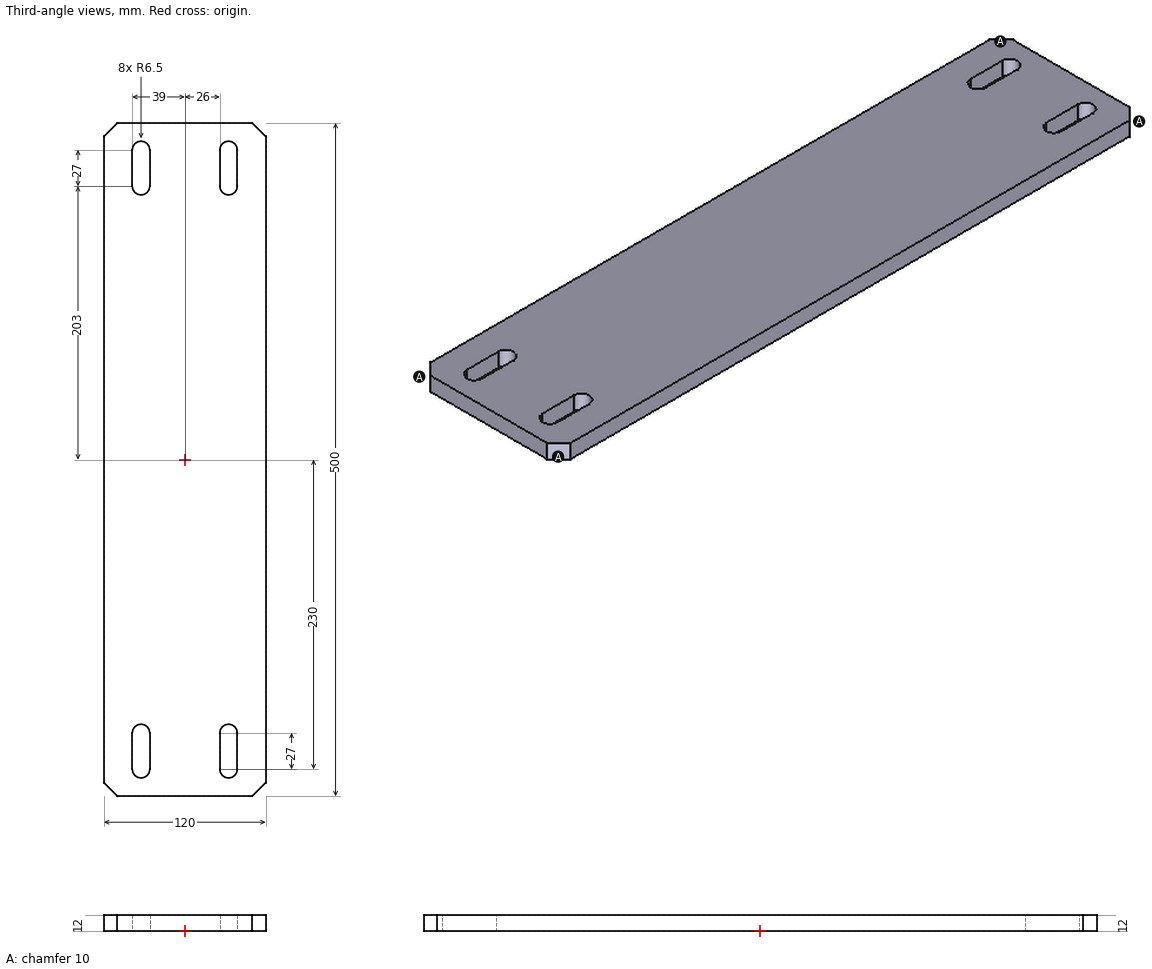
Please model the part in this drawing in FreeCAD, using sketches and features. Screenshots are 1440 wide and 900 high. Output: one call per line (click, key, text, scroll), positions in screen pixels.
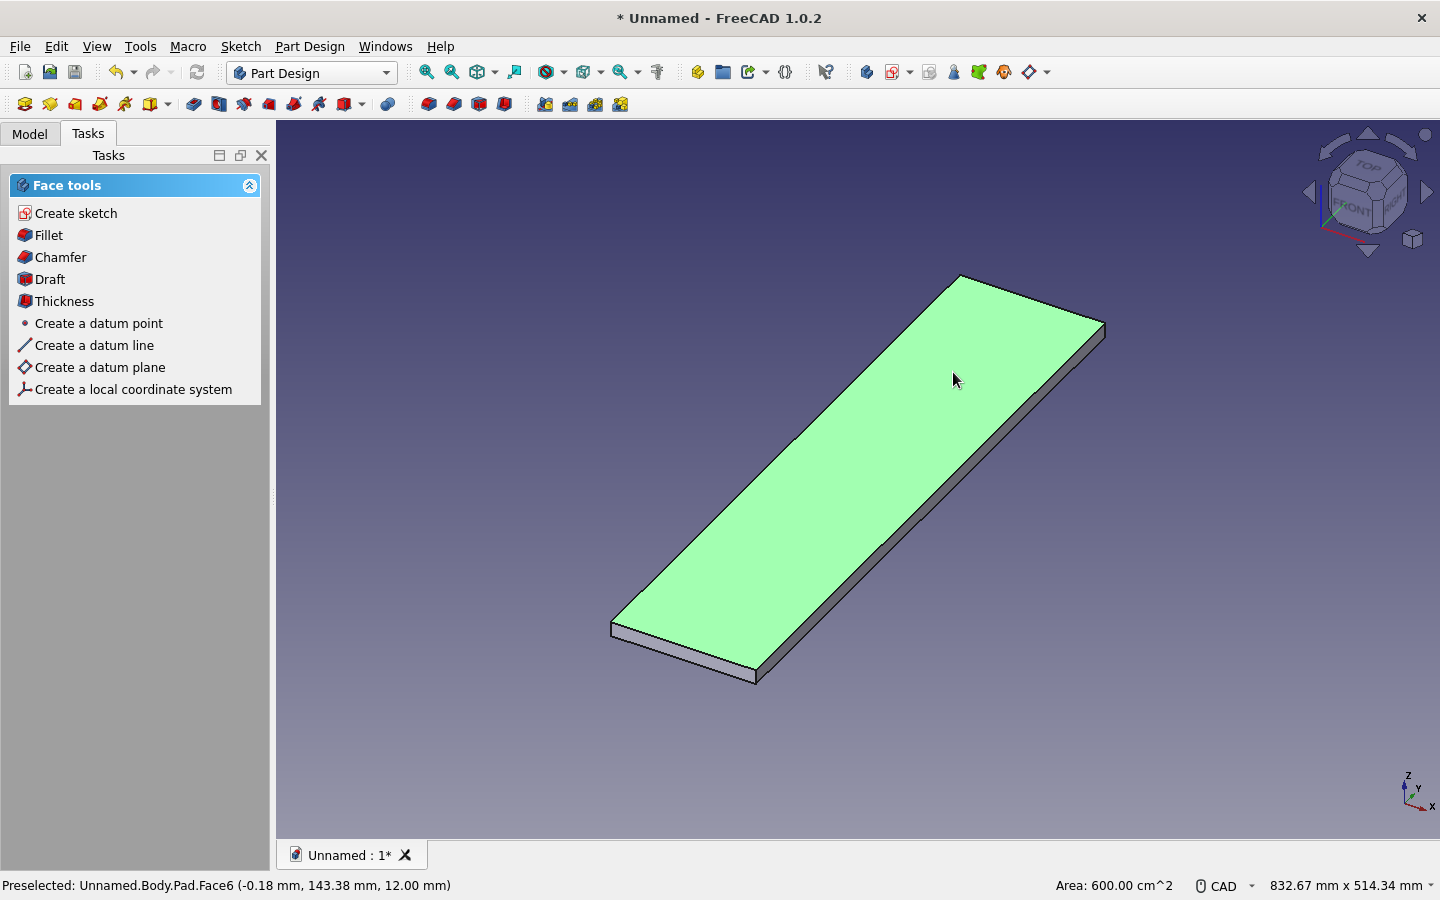
click(892, 72)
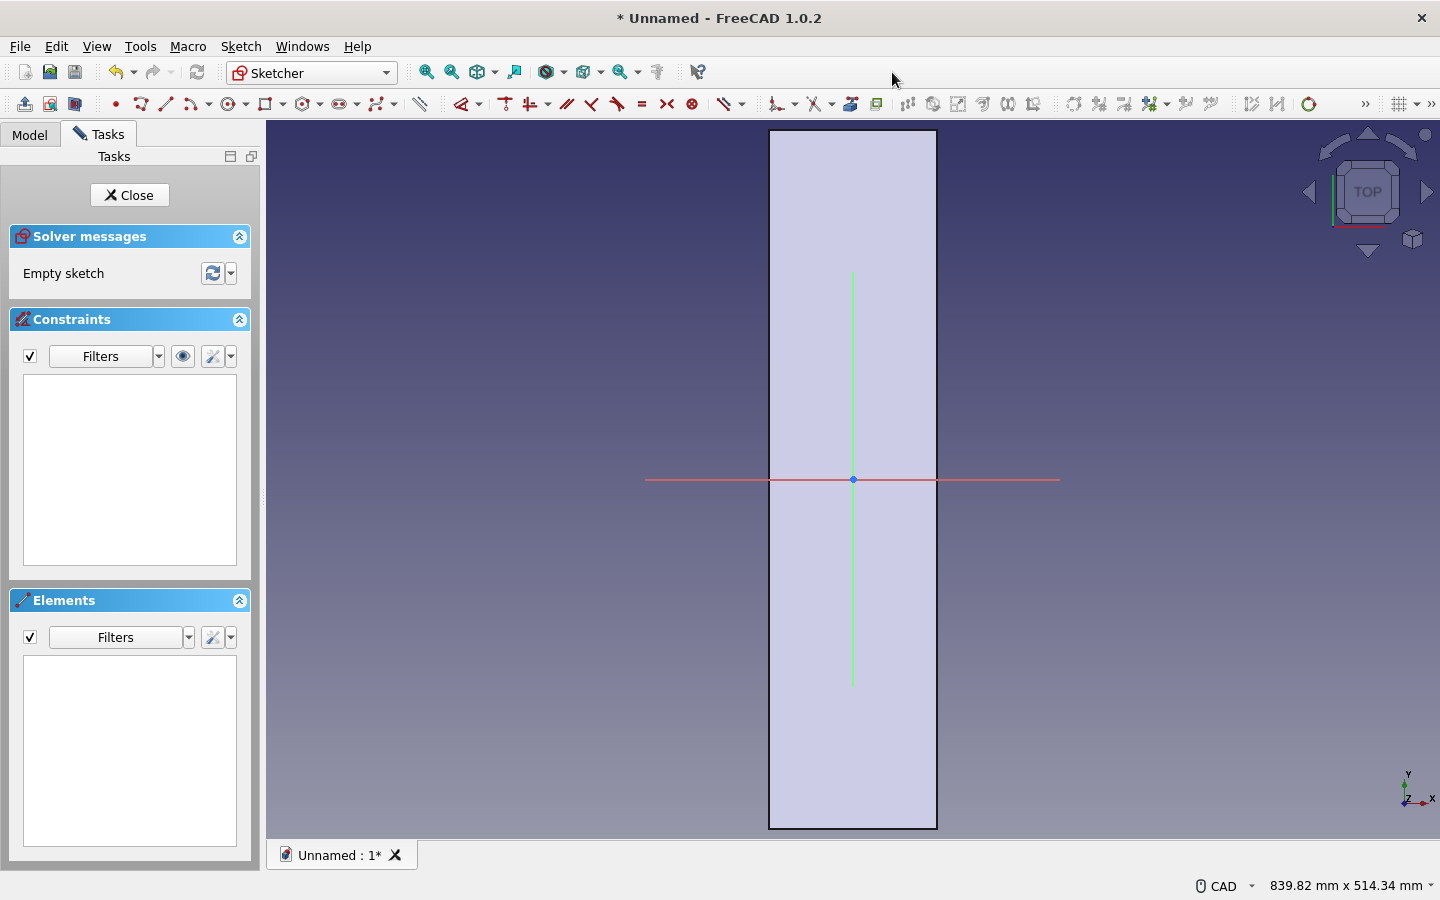
scroll(645, 480, down, 2)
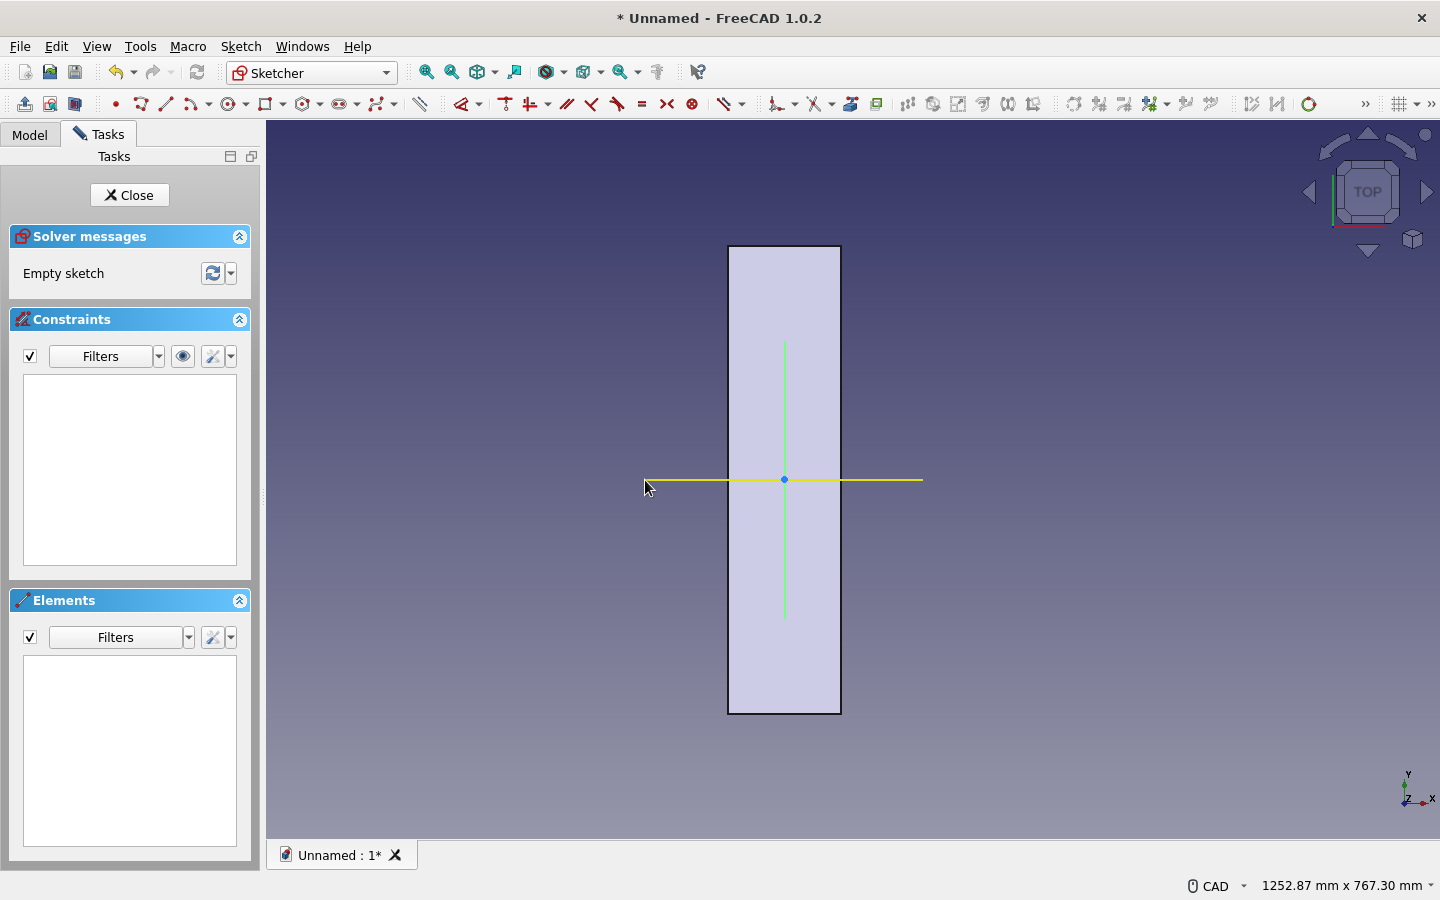
key(g)
key(s)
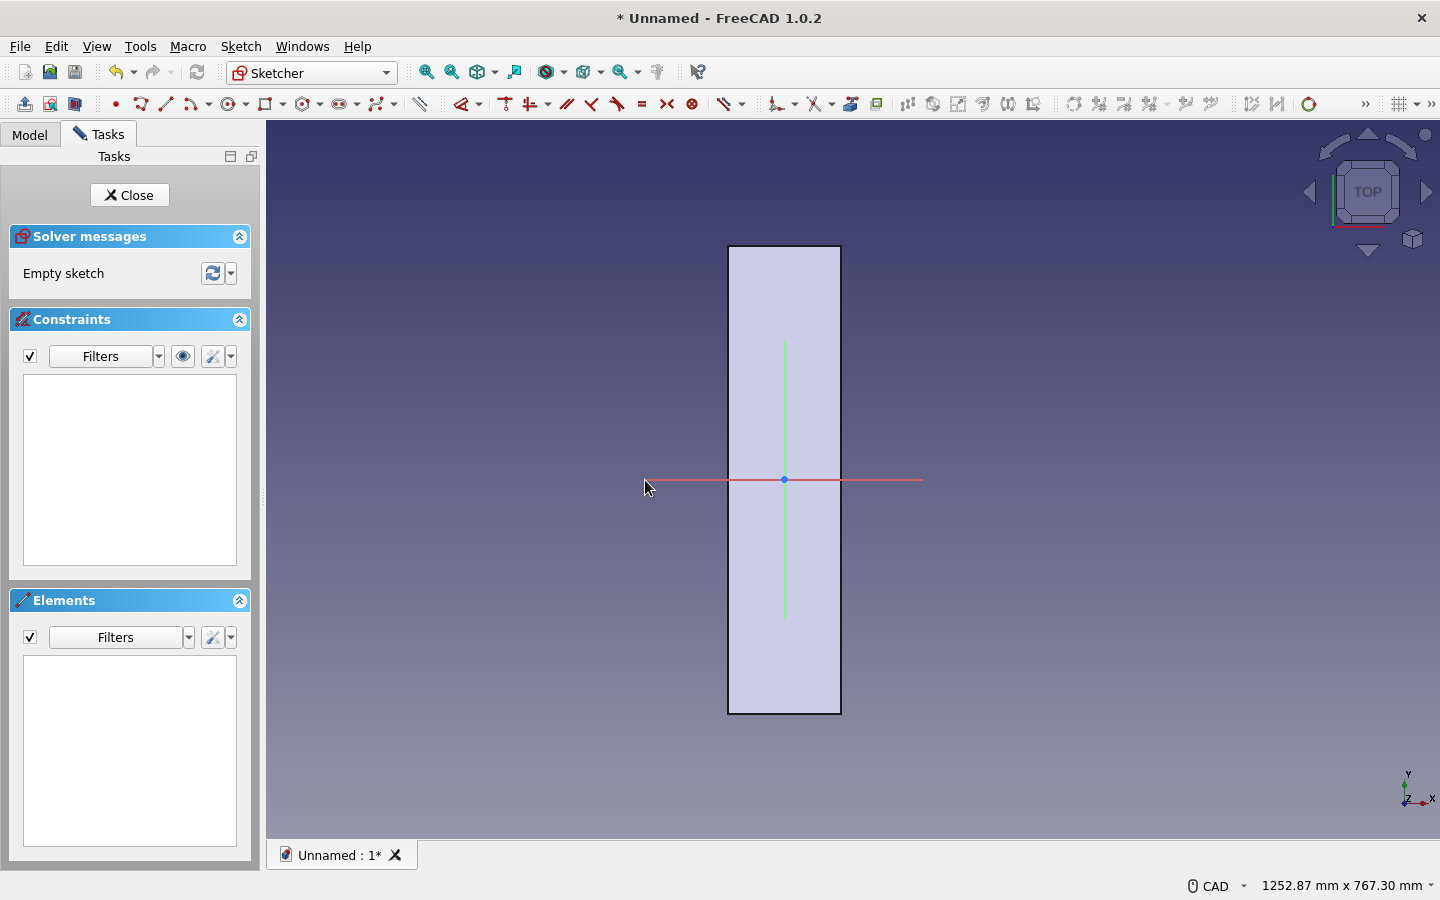
scroll(754, 290, up, 7)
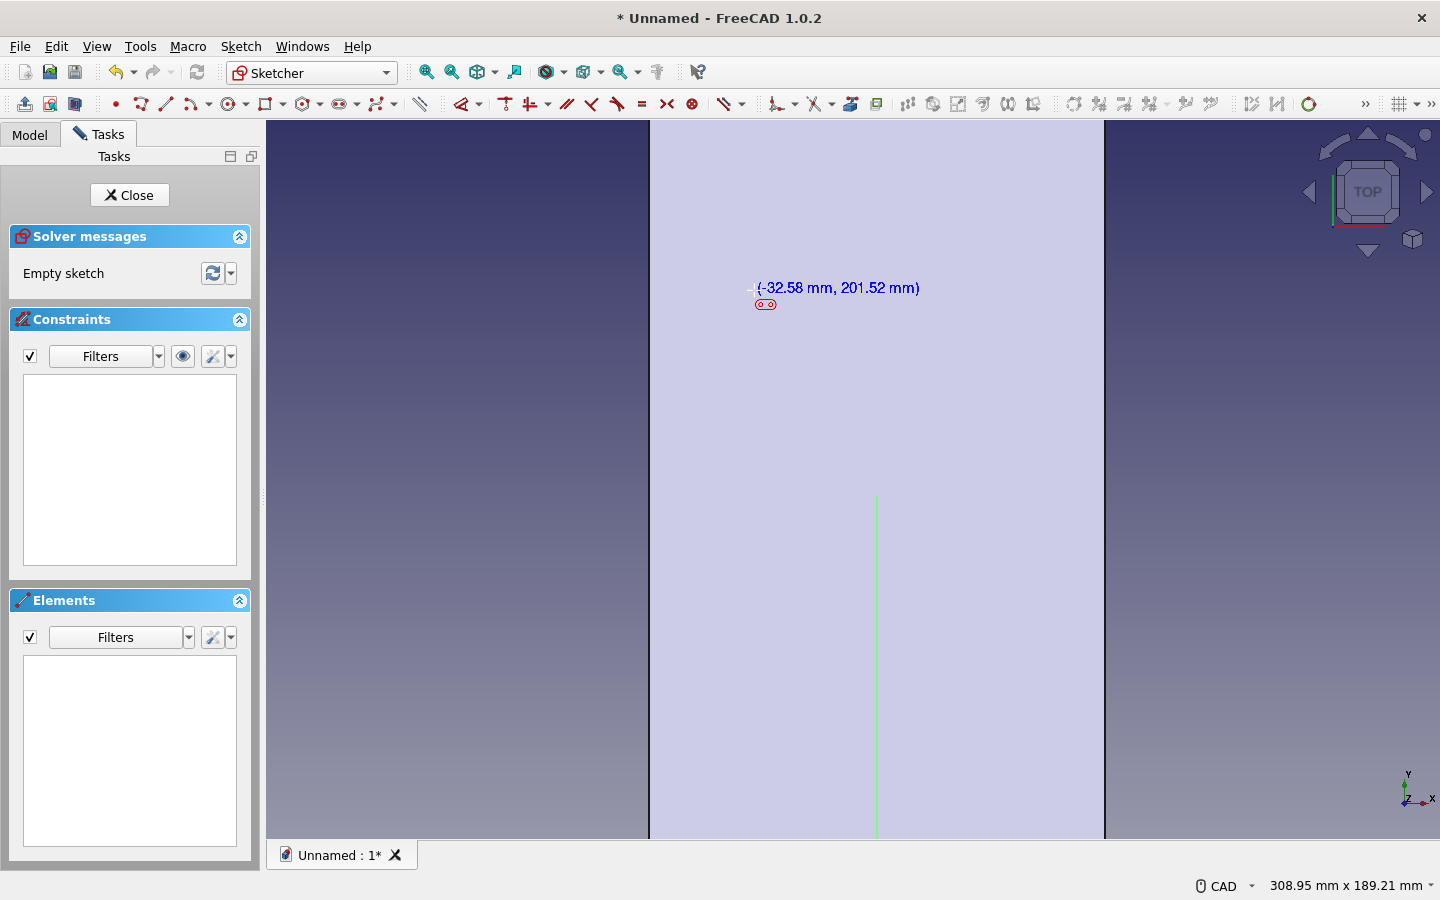
scroll(754, 290, down, 7)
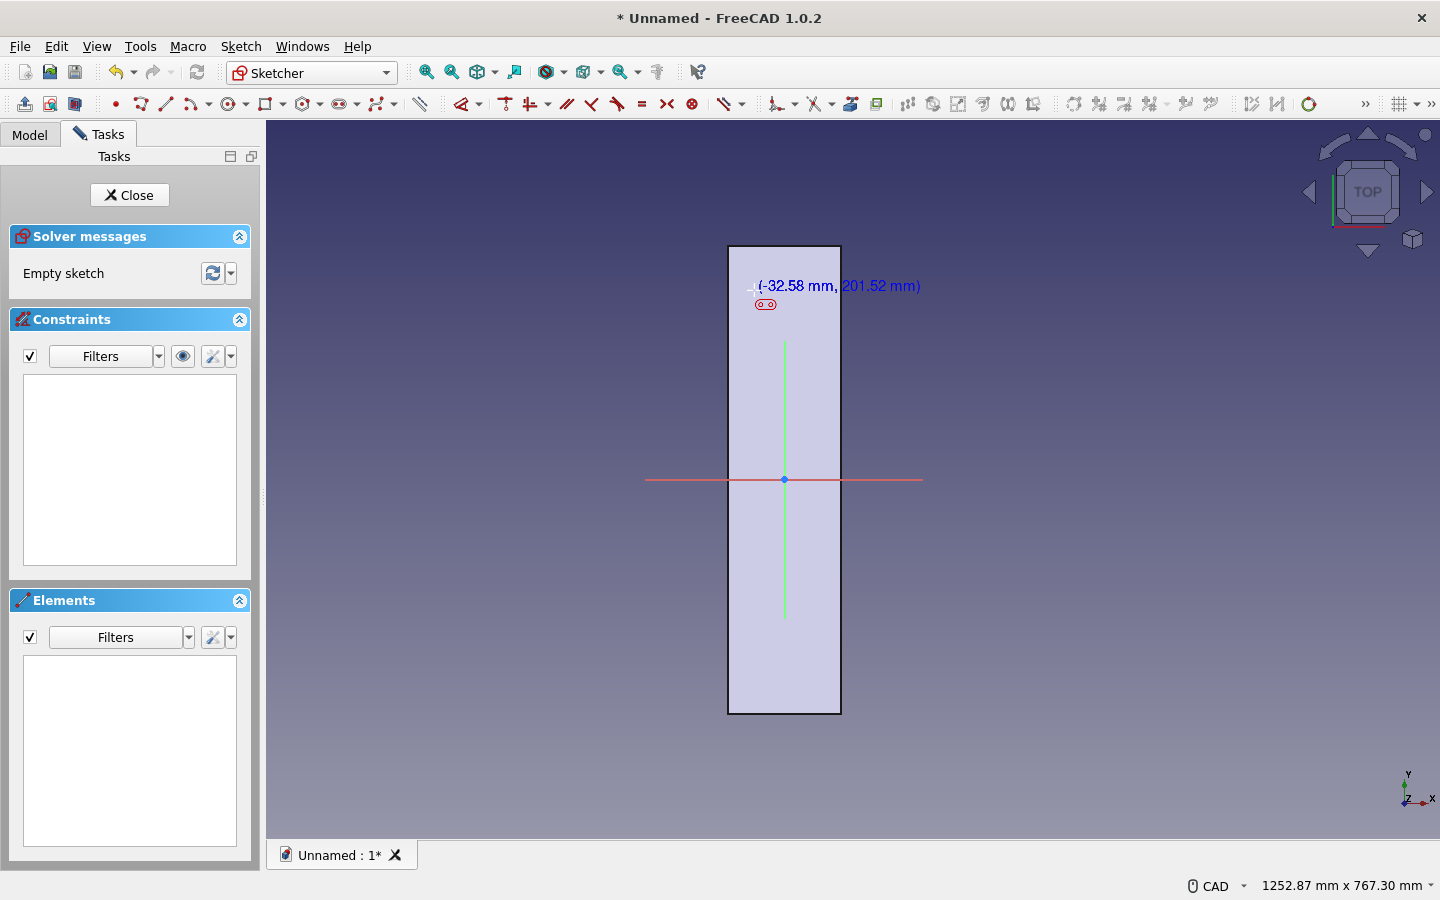
click(754, 290)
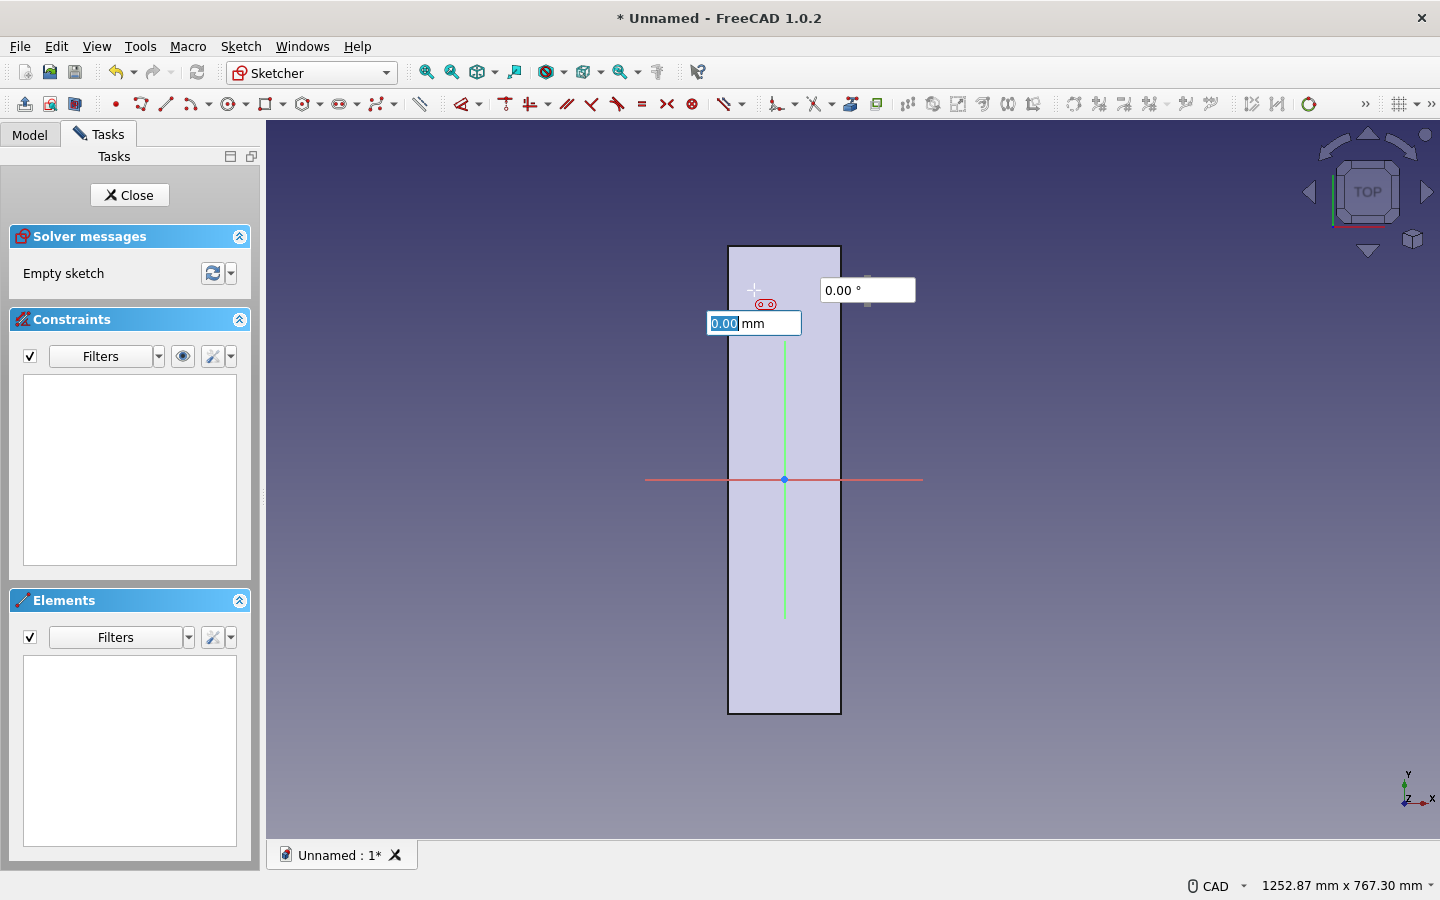
click(754, 264)